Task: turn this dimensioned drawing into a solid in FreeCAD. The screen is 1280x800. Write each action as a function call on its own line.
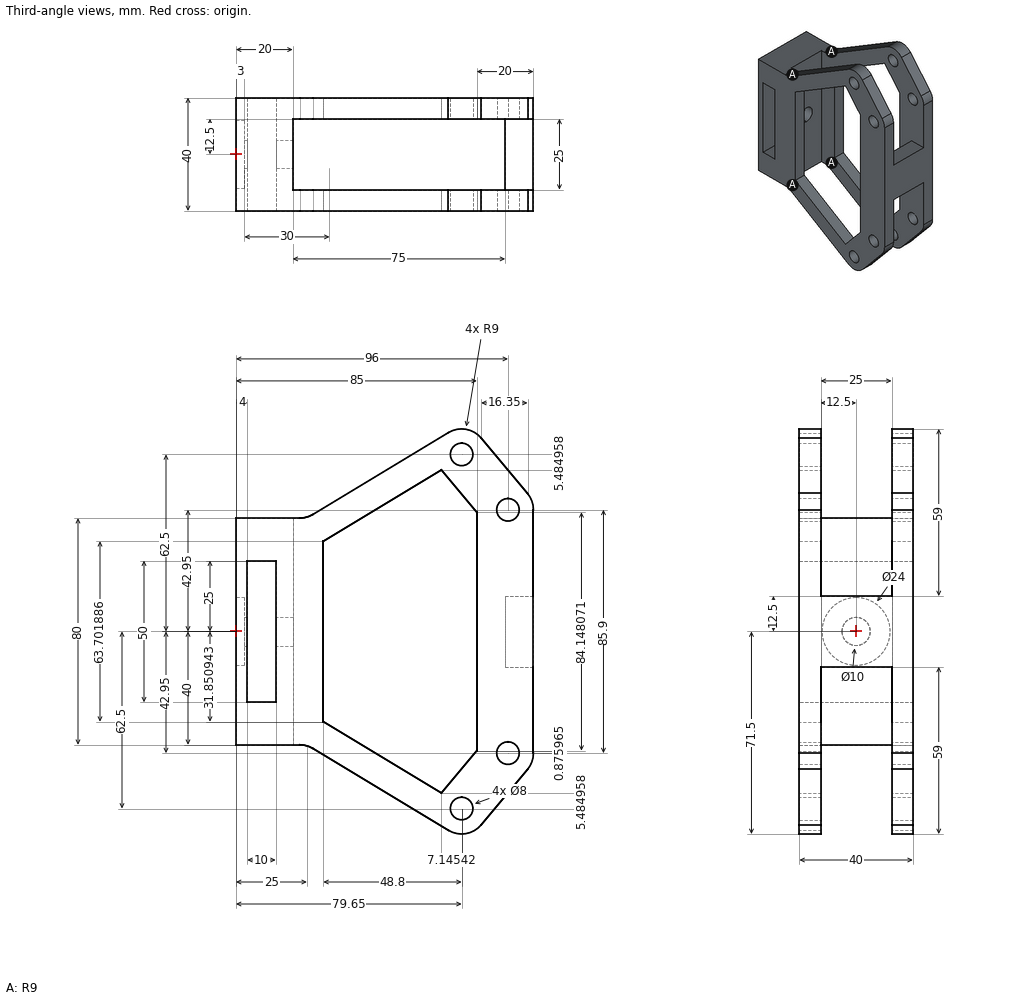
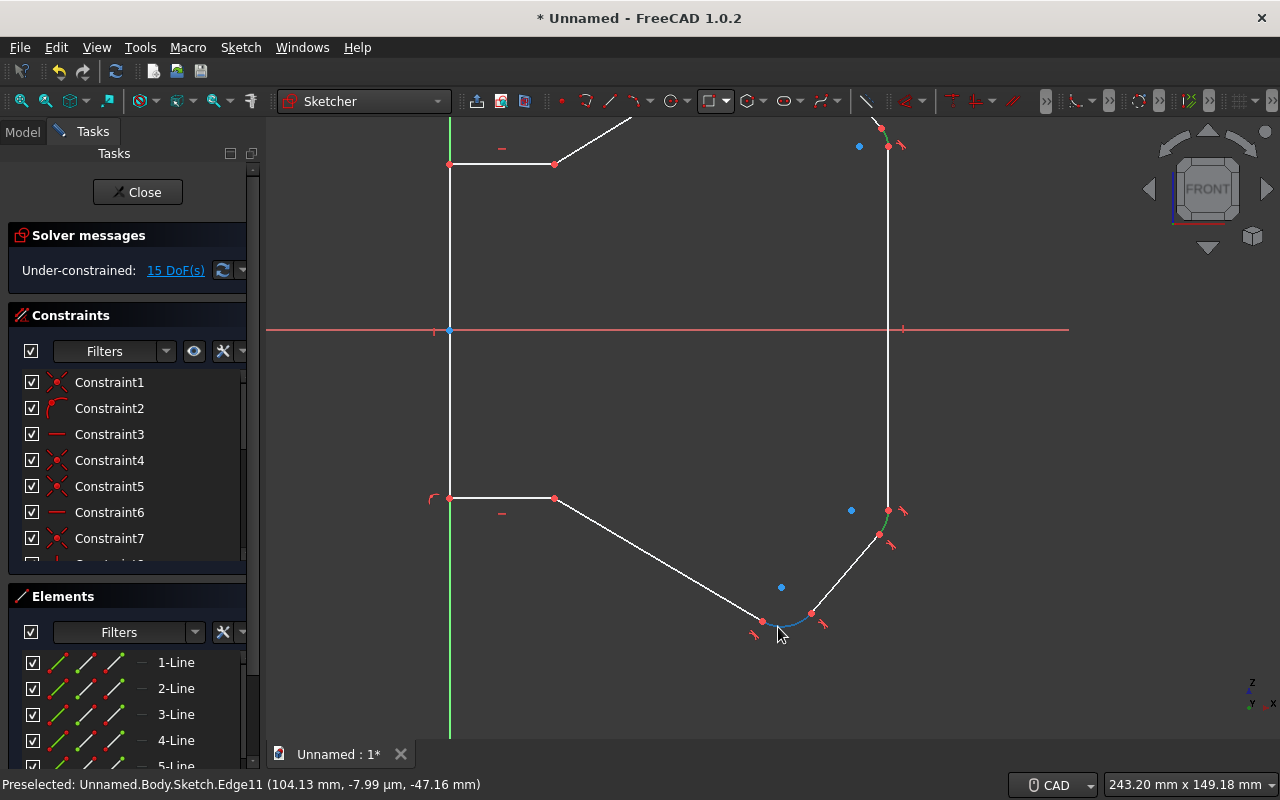
click(777, 626)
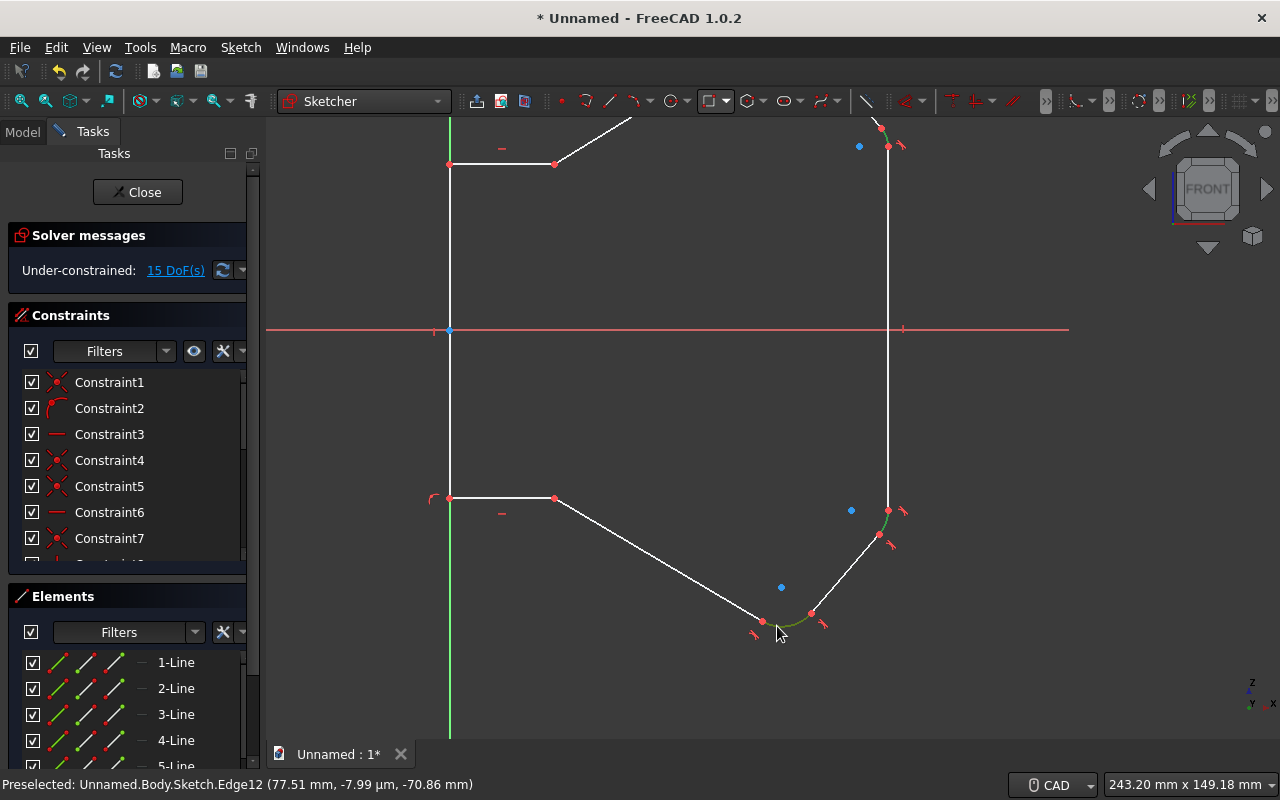
key(e)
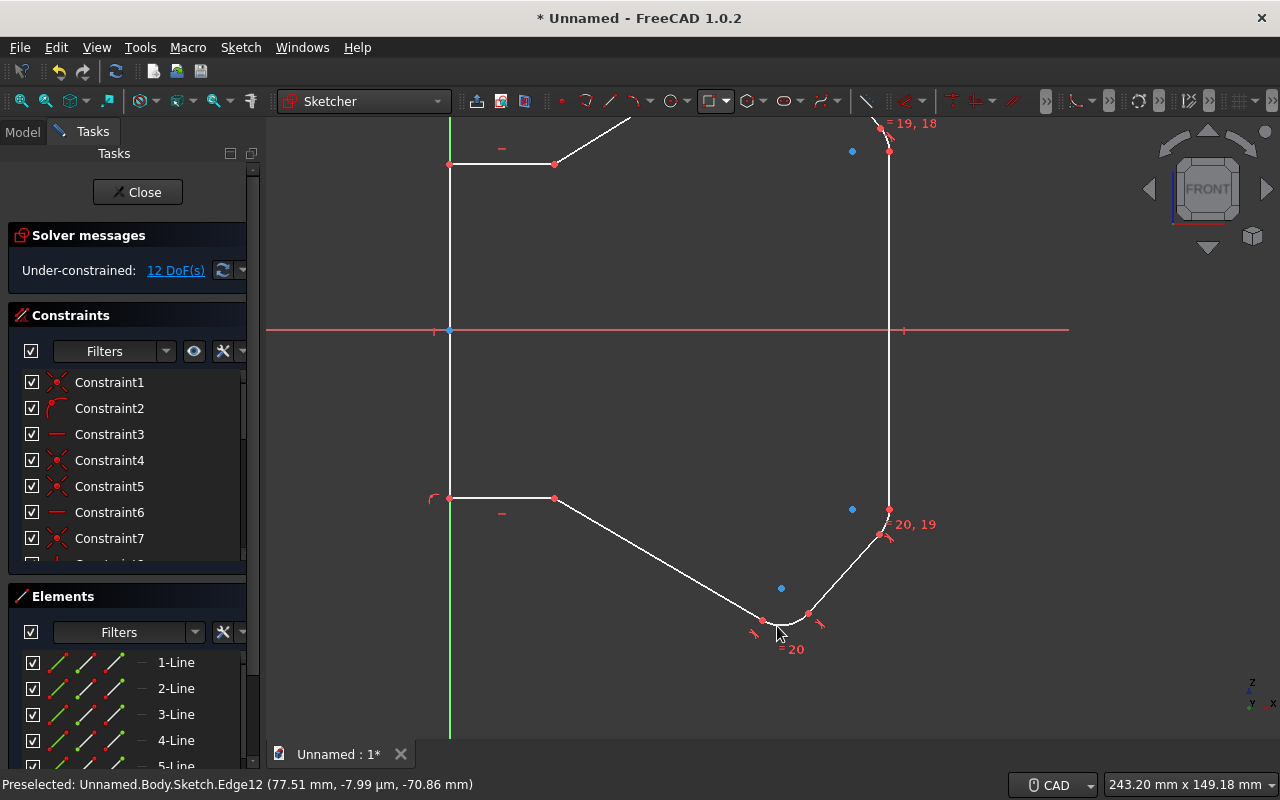
scroll(777, 627, down, 2)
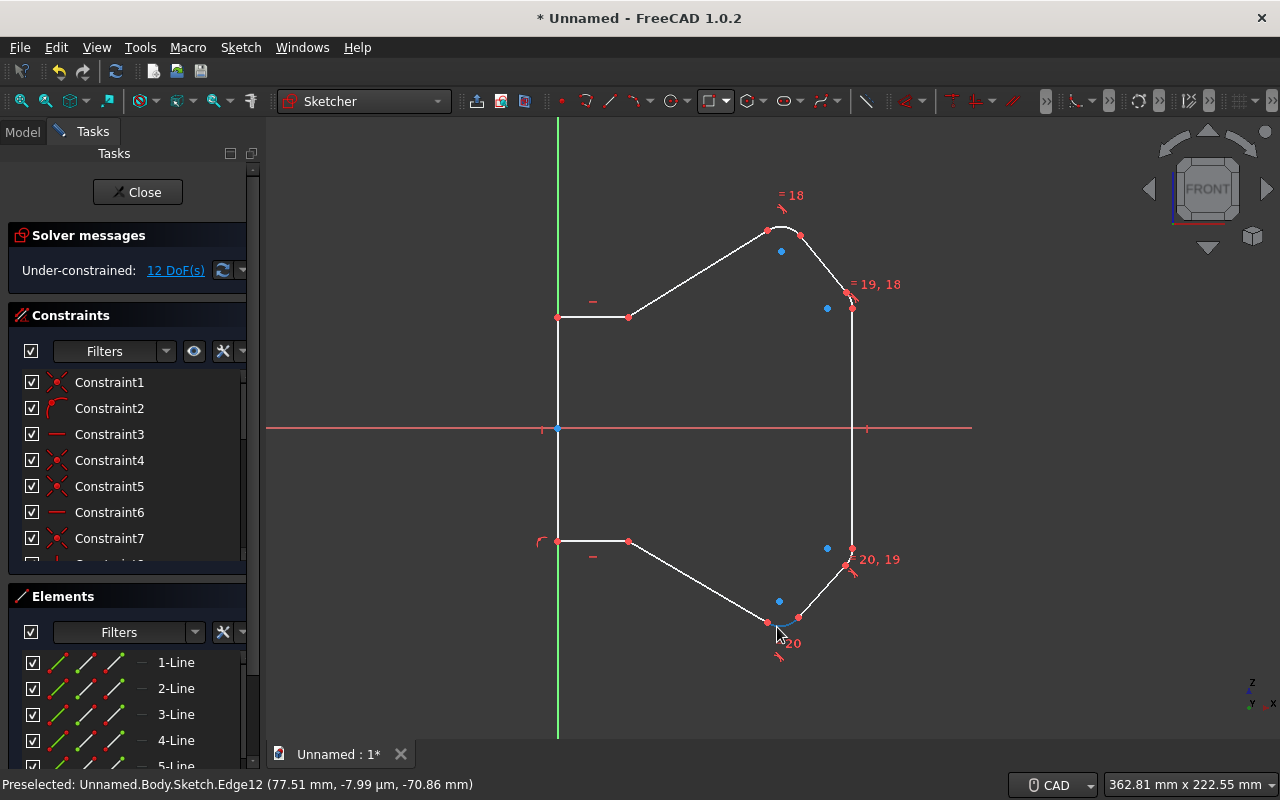
scroll(792, 229, up, 3)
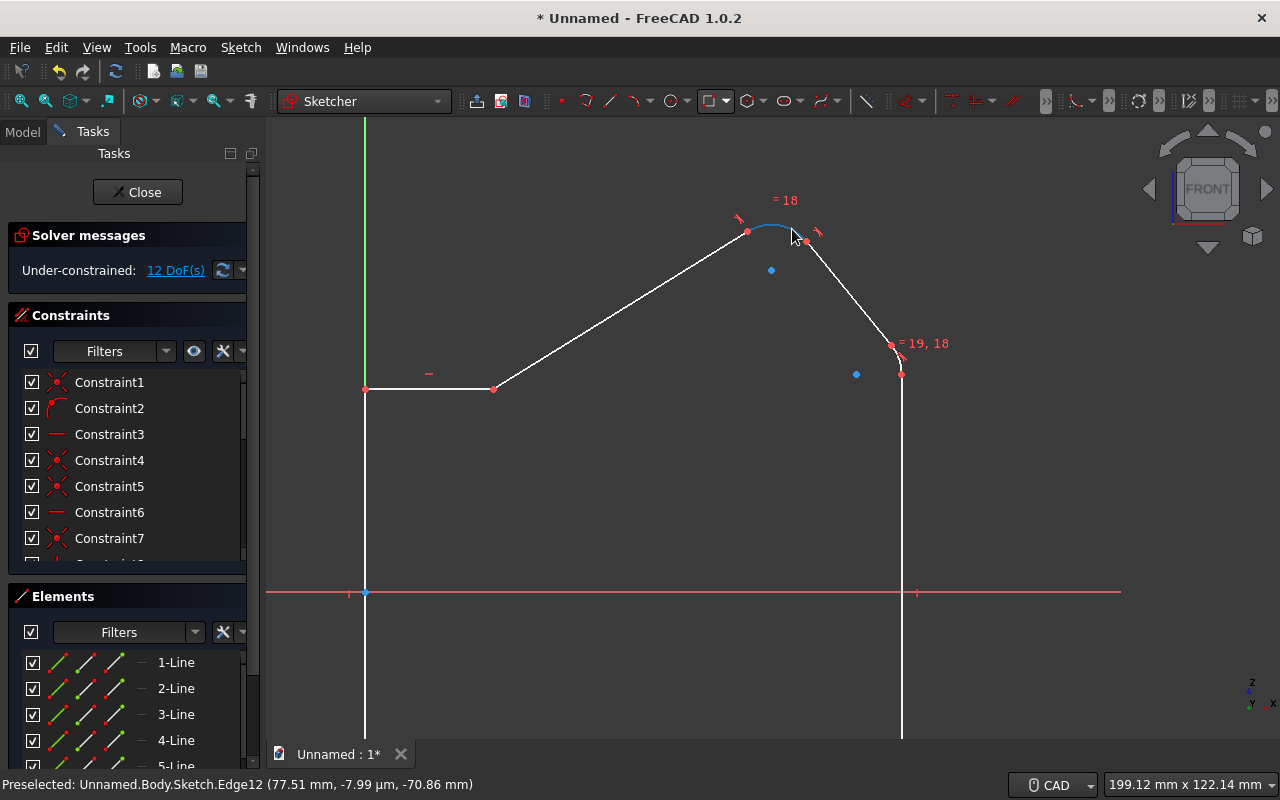
click(792, 229)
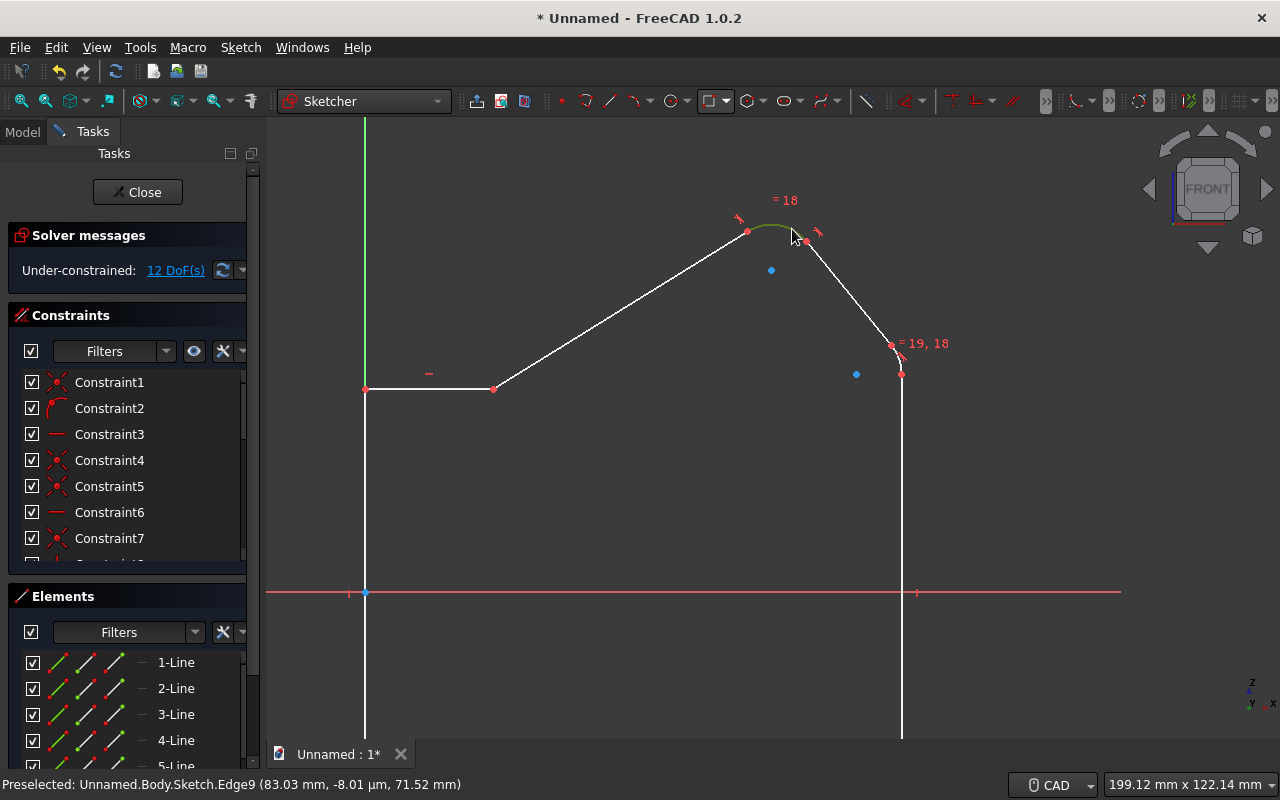
key(k)
key(r)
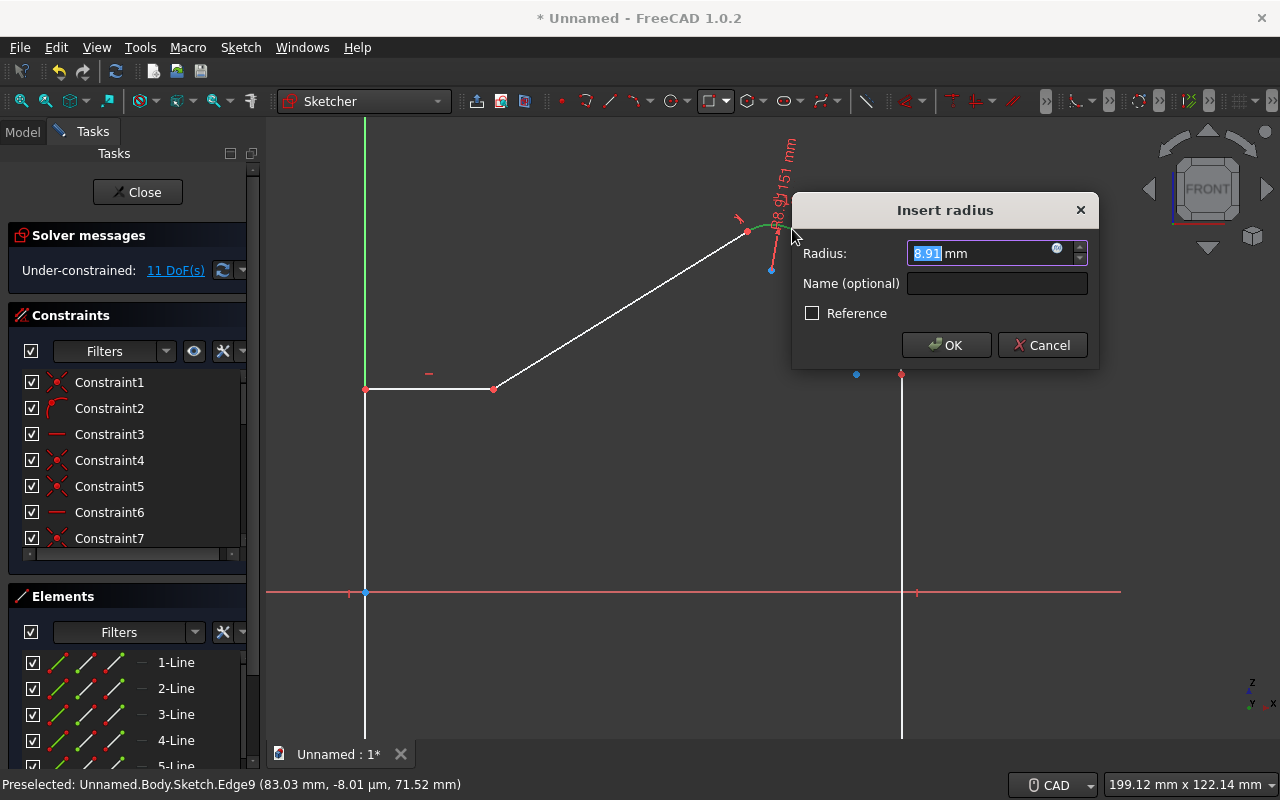
text(9)
key(Return)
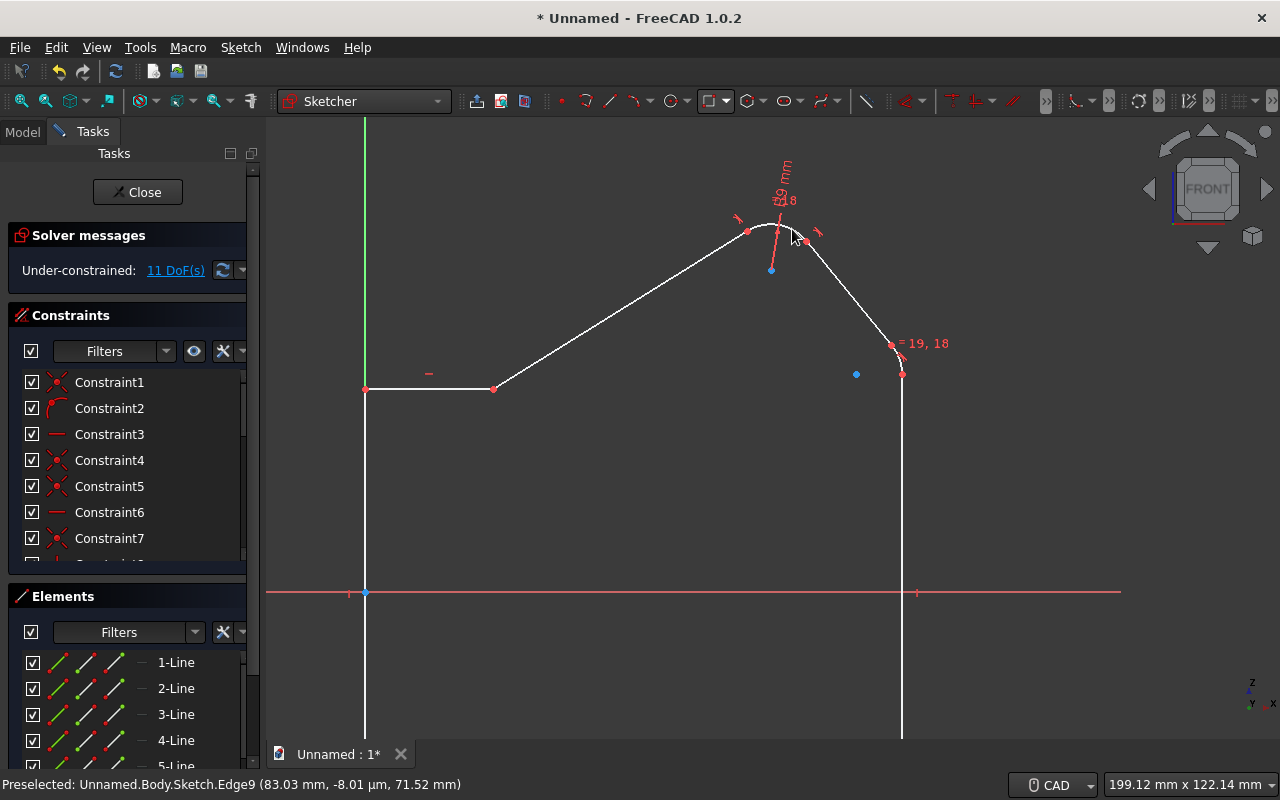
scroll(792, 228, down, 3)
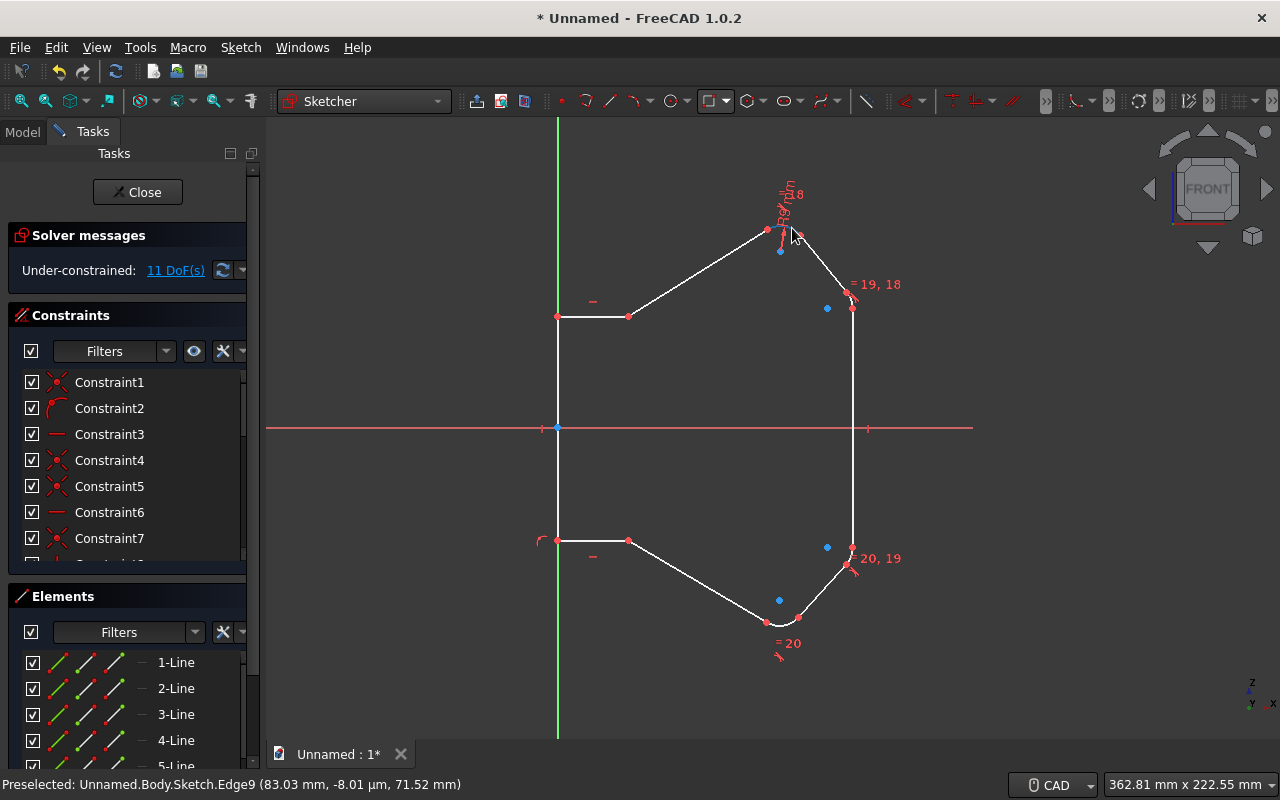
click(607, 541)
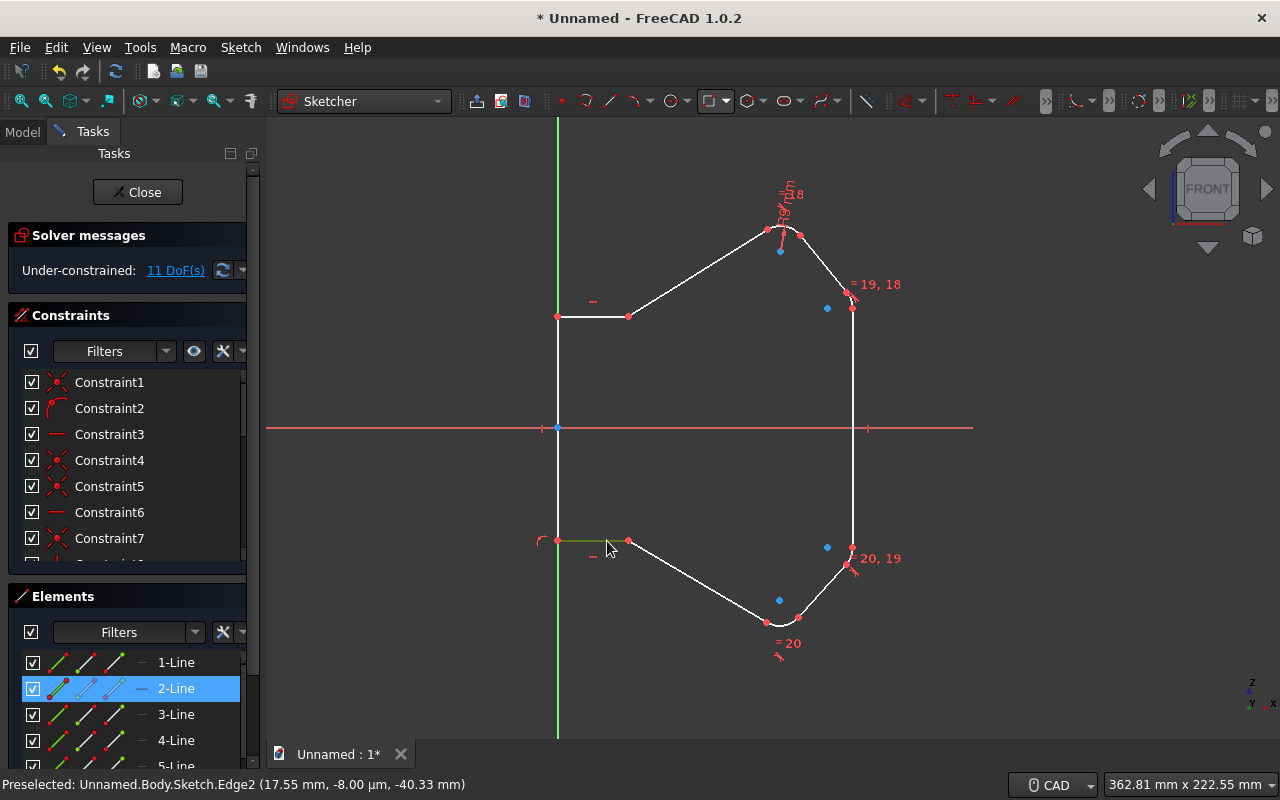
key(l)